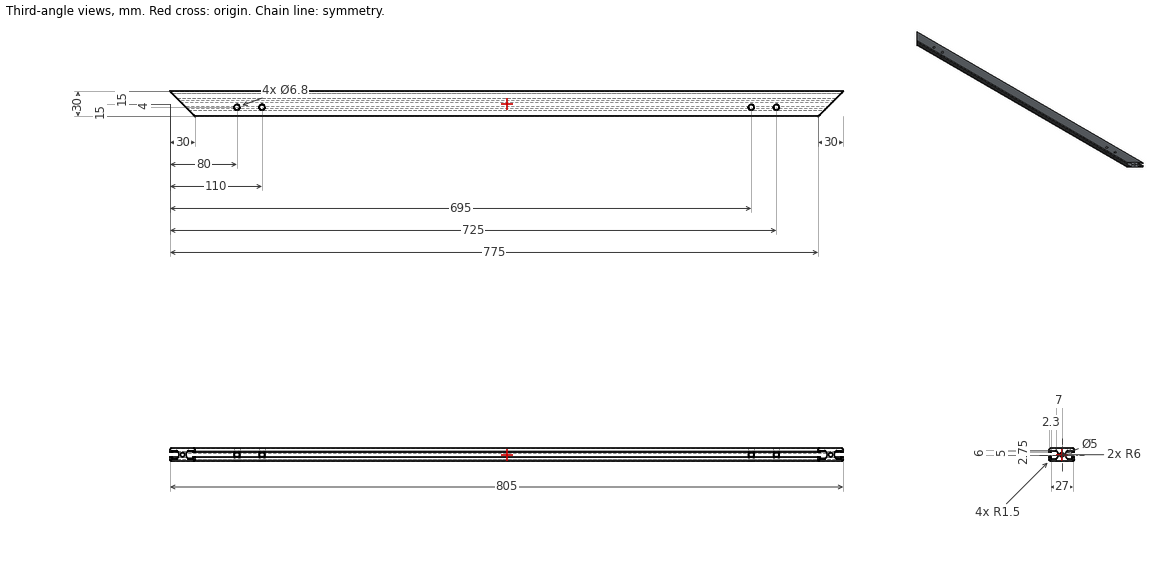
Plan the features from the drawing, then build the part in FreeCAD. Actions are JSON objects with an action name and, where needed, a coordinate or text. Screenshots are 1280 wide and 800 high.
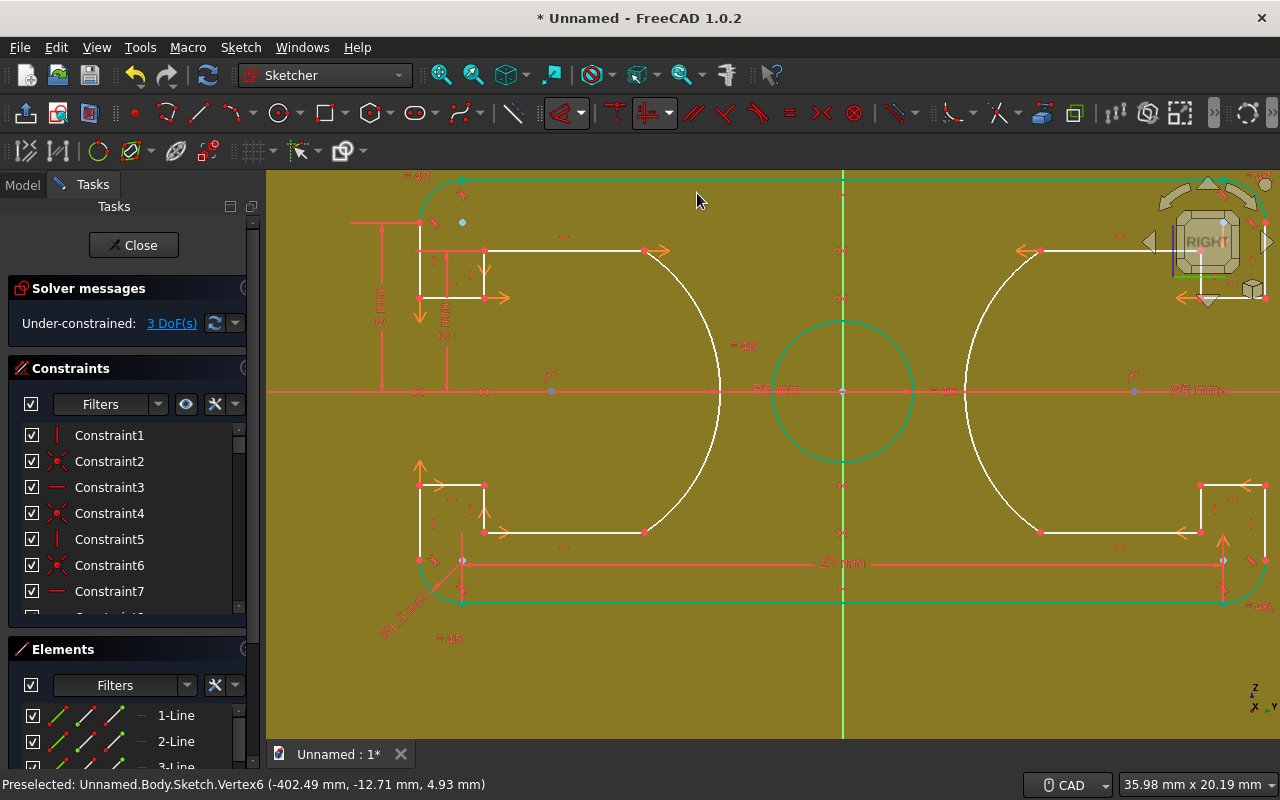
{"action": "left_click", "coordinate": [645, 251]}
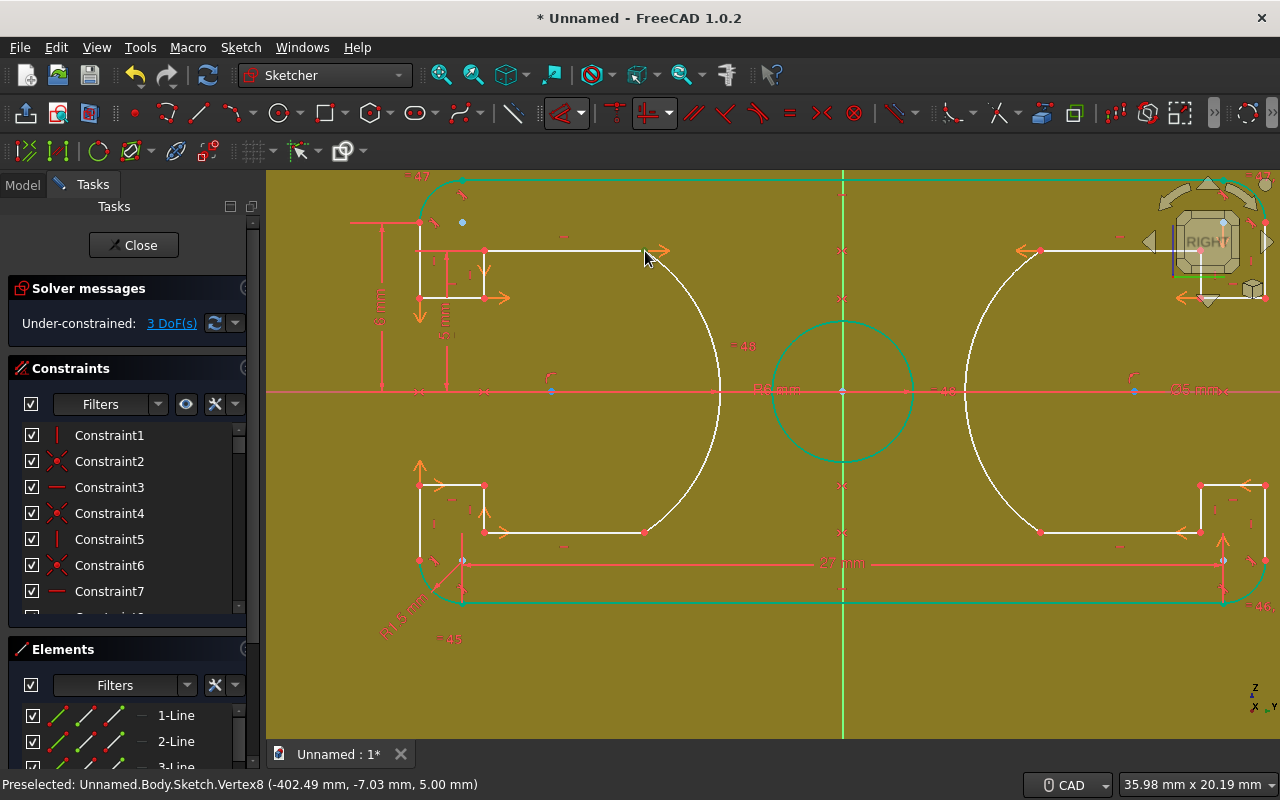
{"action": "left_click", "coordinate": [584, 114]}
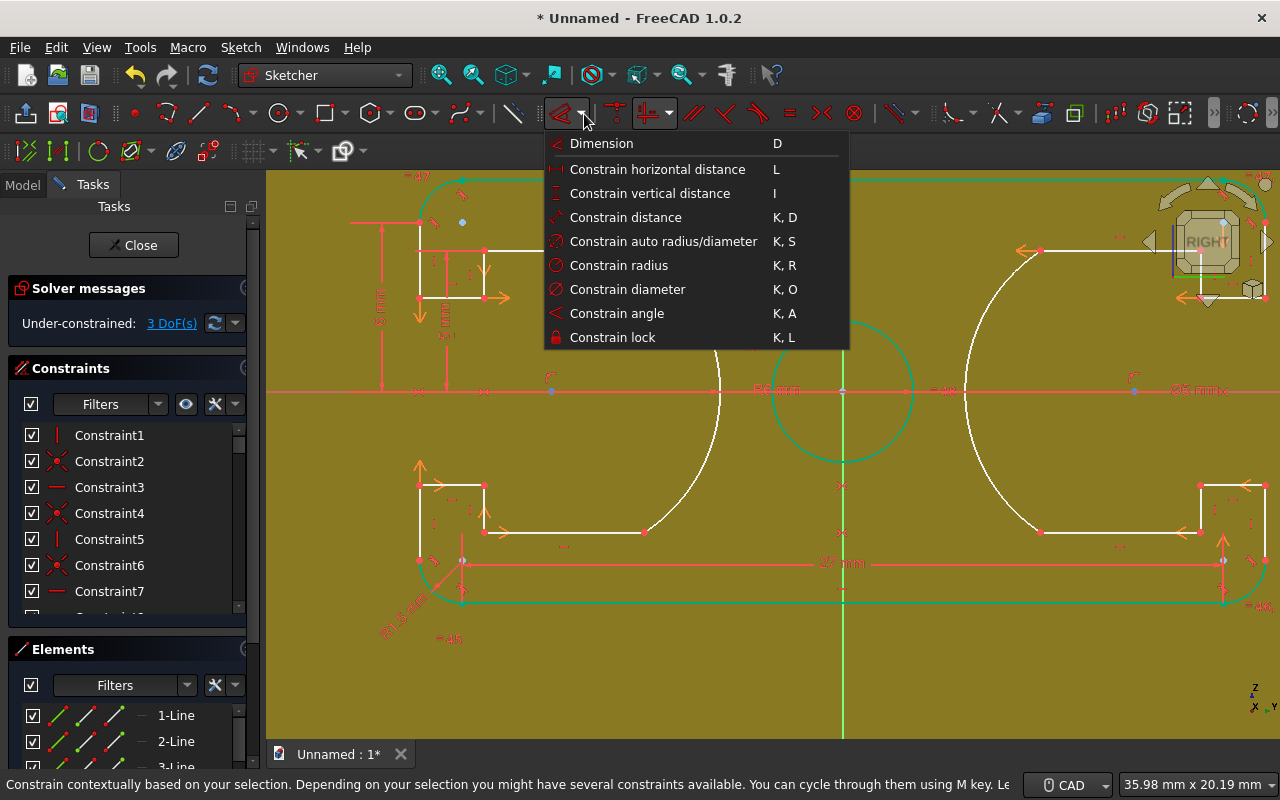
{"action": "left_click", "coordinate": [697, 169]}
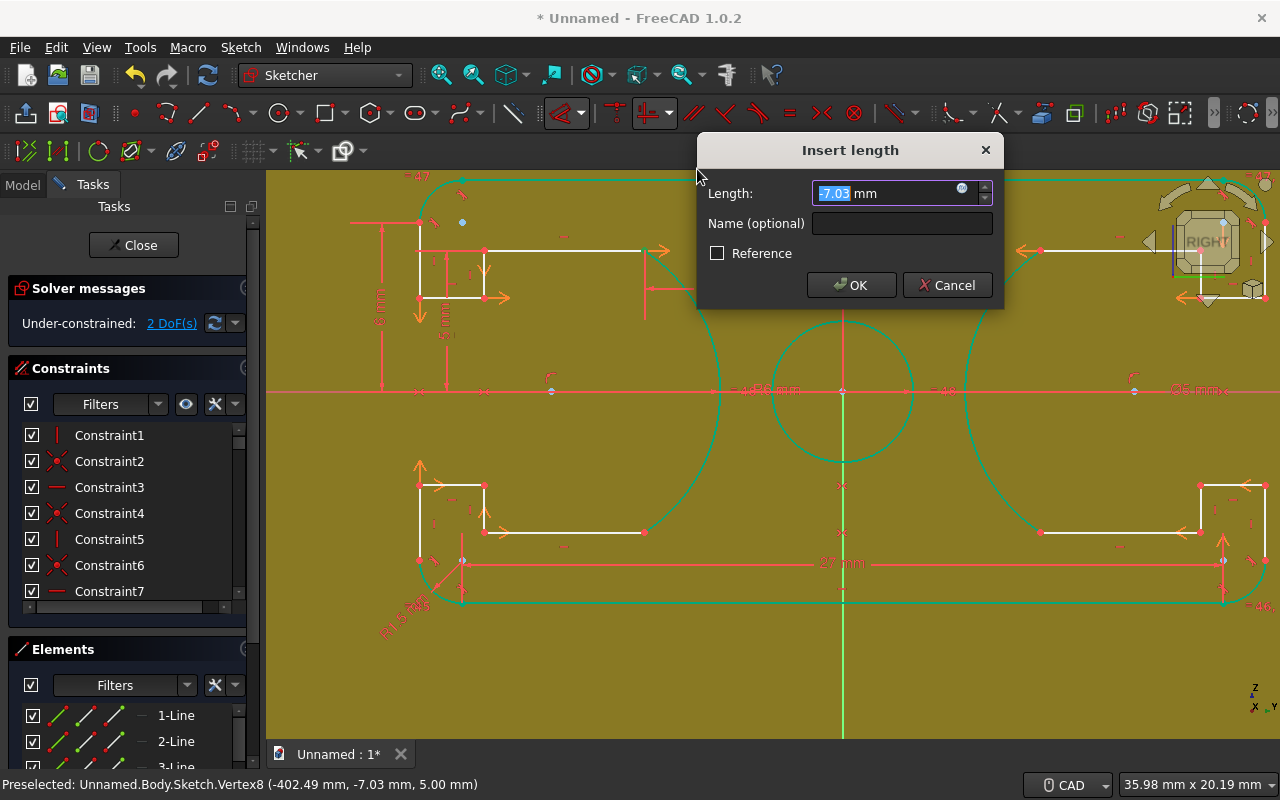
{"action": "type", "text": "-7"}
{"action": "key", "text": "Return"}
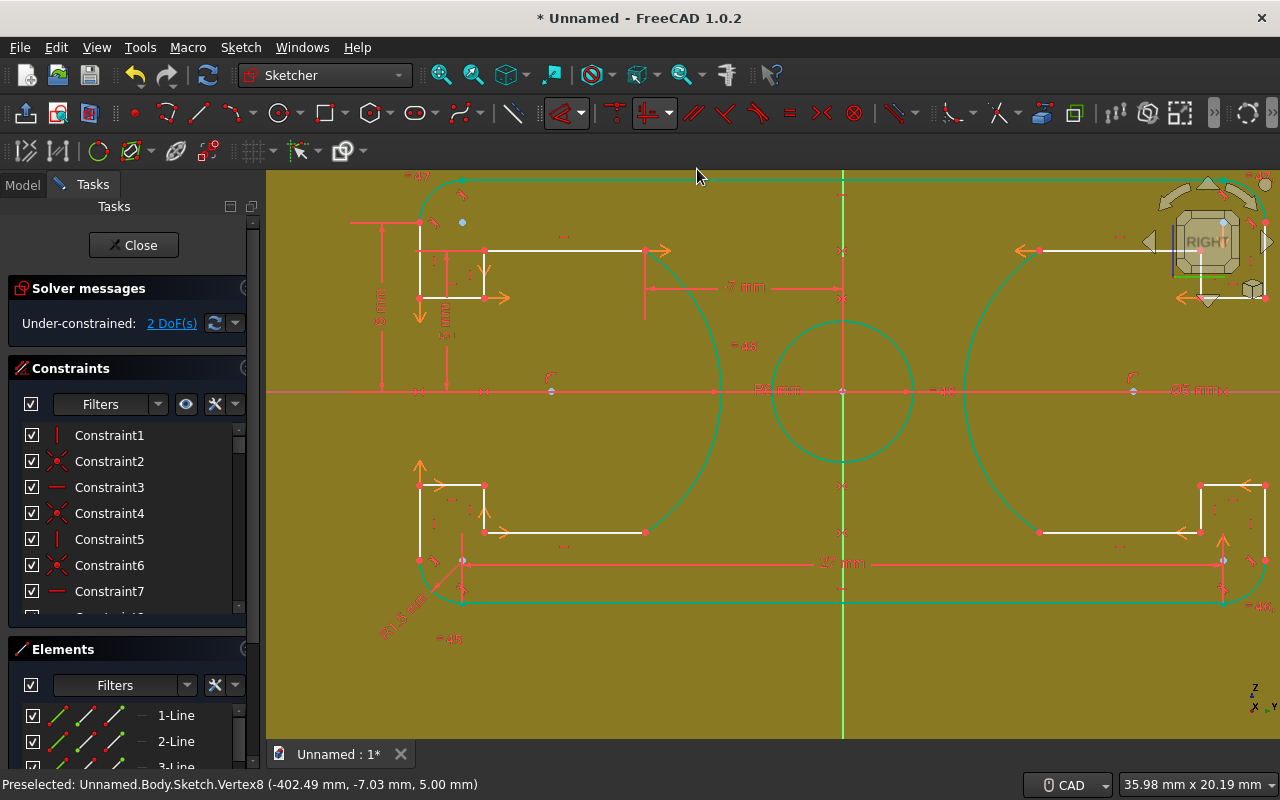
{"action": "left_click", "coordinate": [439, 298]}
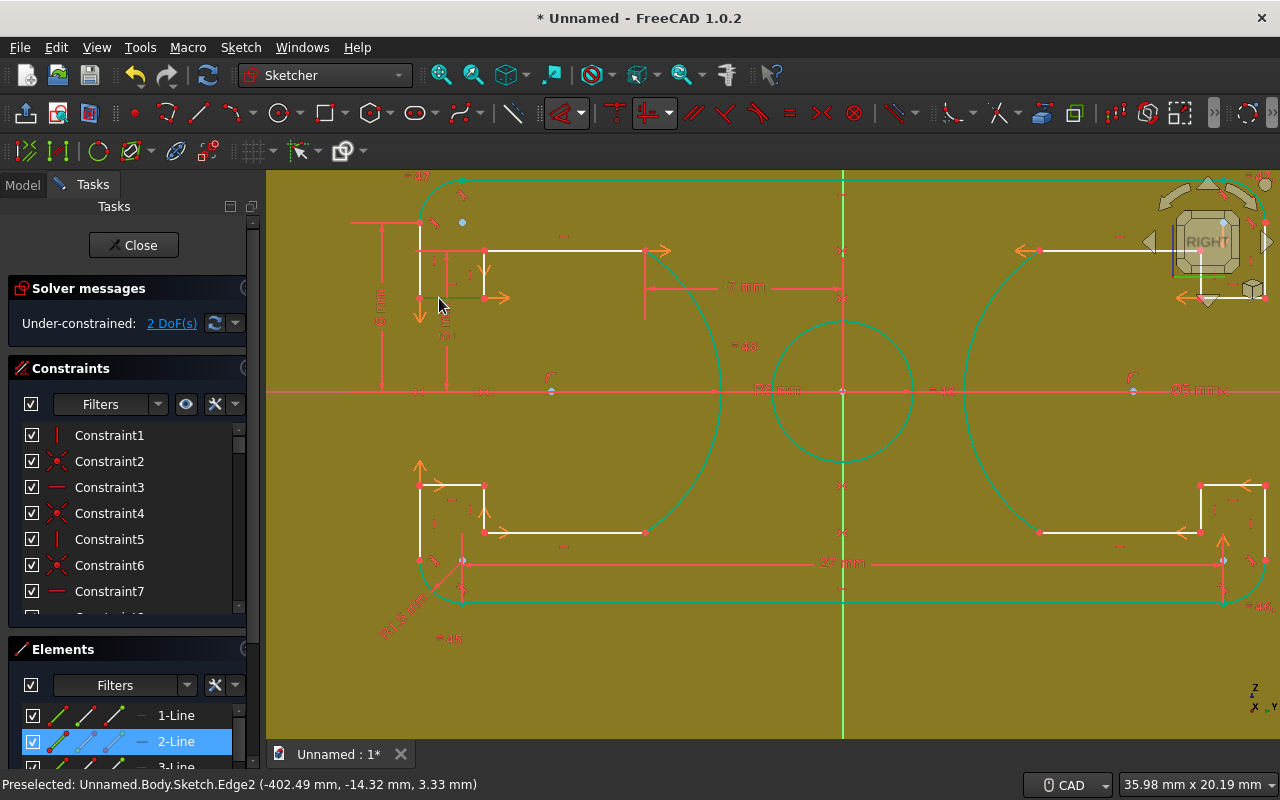
{"action": "left_click", "coordinate": [584, 114]}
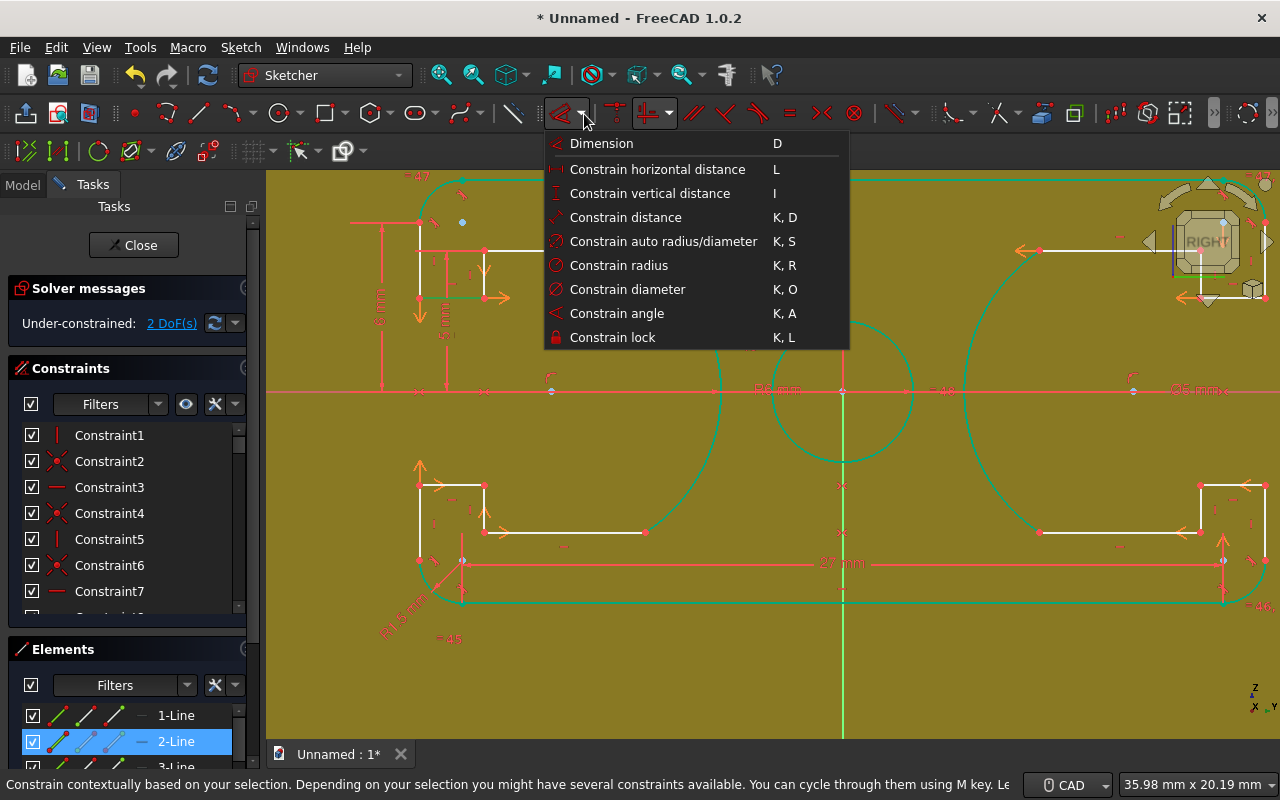
{"action": "left_click", "coordinate": [697, 169]}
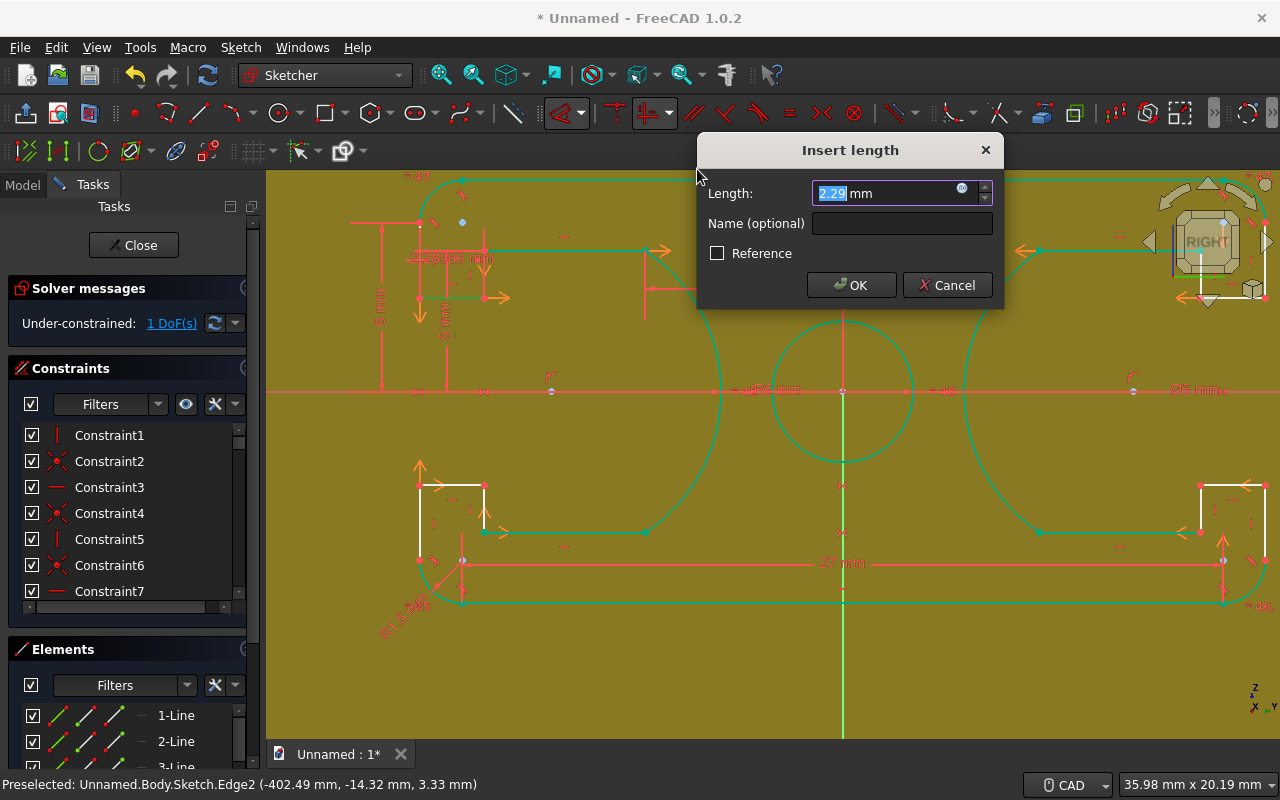
{"action": "type", "text": "2.3"}
{"action": "key", "text": "Return"}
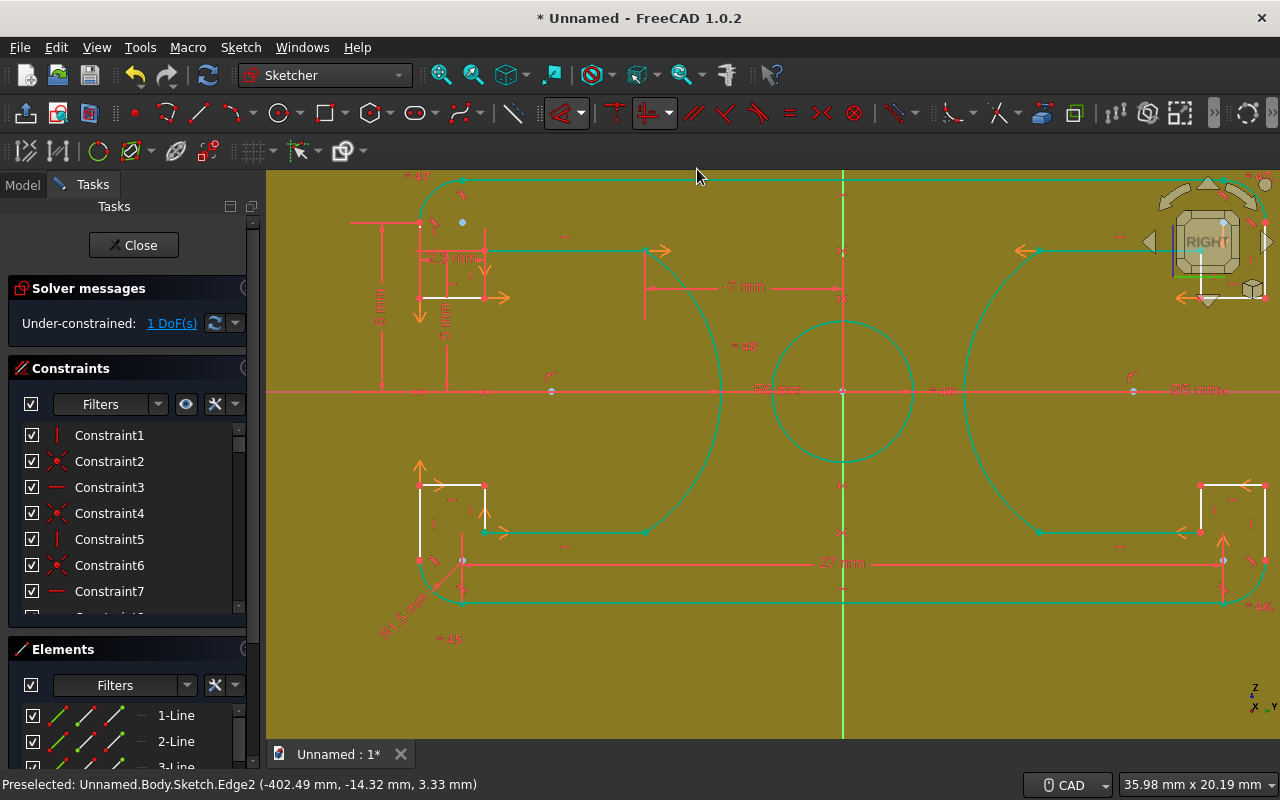
{"action": "left_click", "coordinate": [420, 245]}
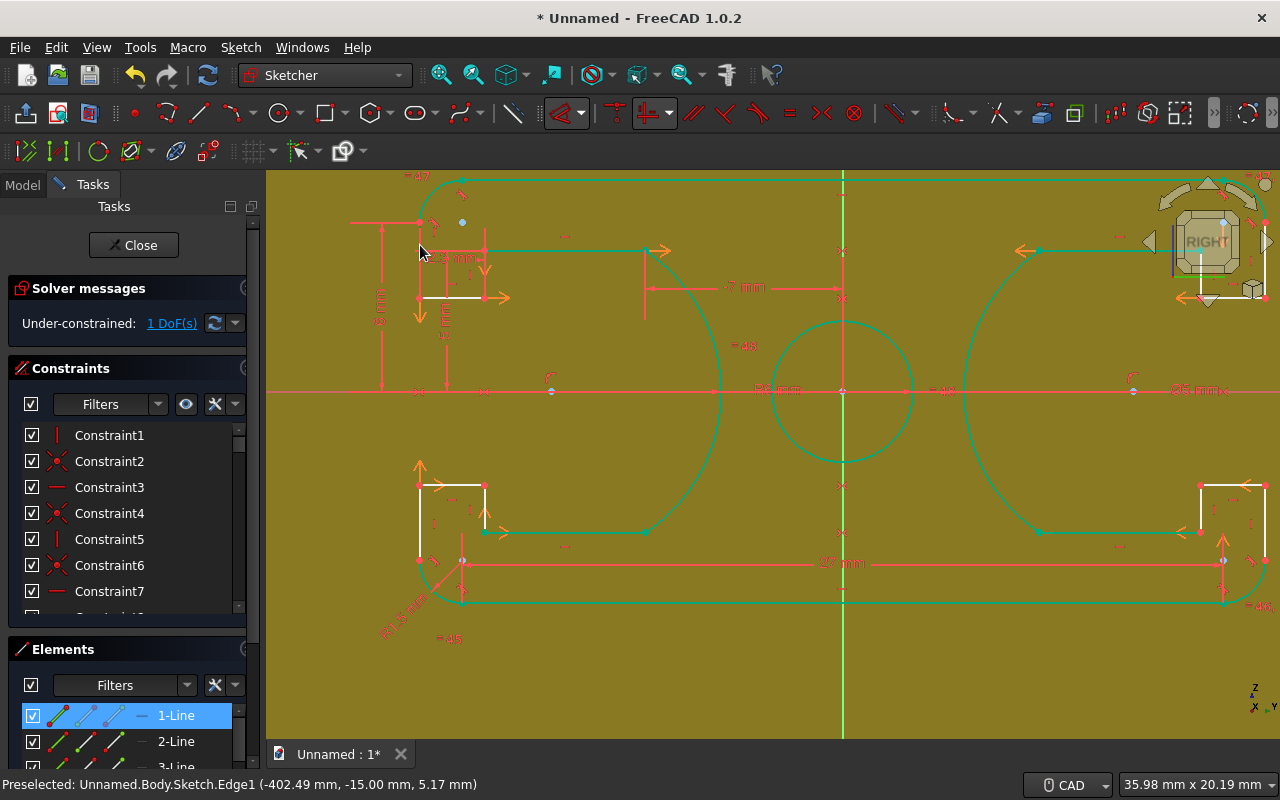
{"action": "left_click", "coordinate": [584, 114]}